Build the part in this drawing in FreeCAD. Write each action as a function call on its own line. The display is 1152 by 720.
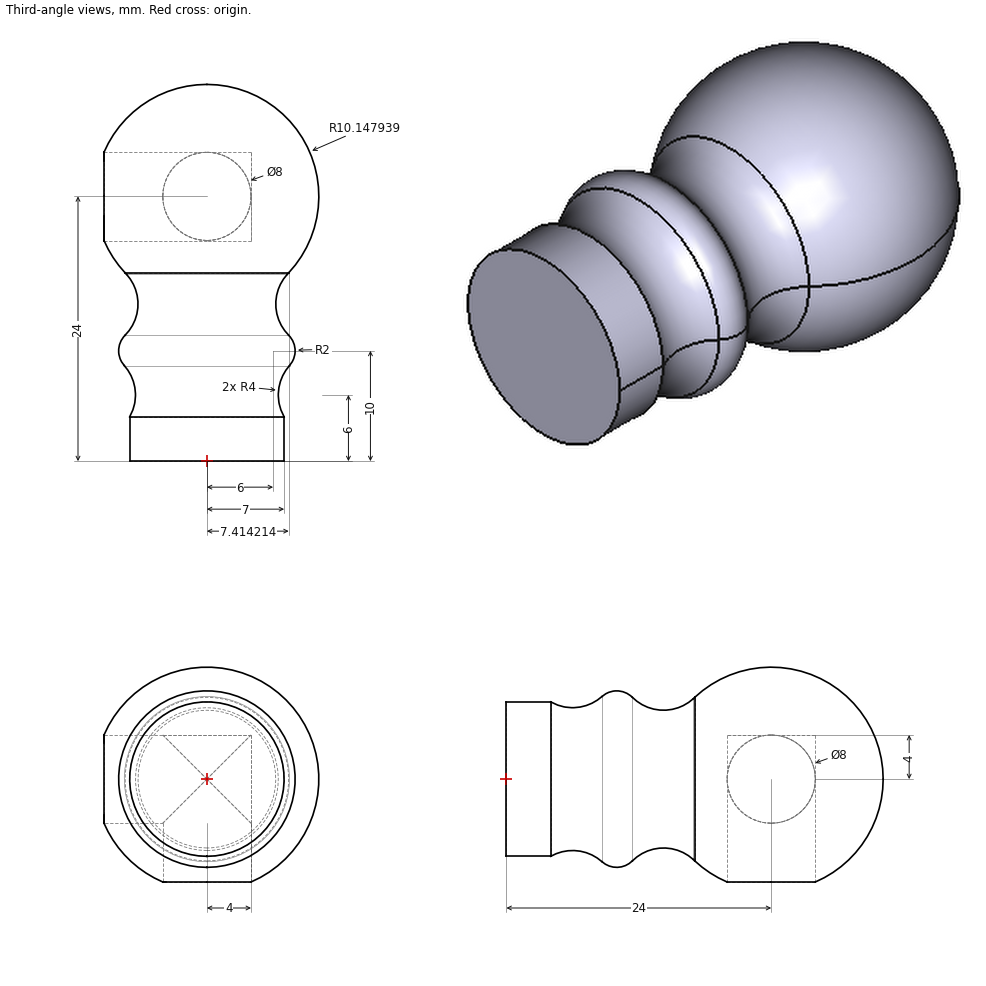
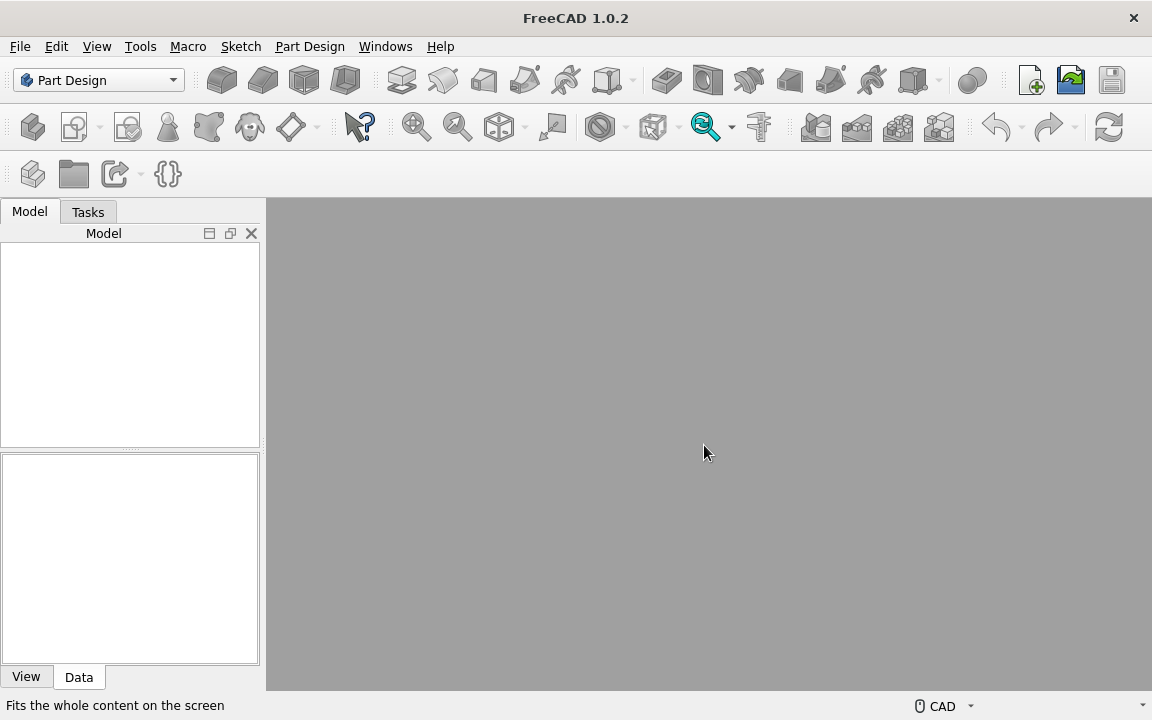
click(1030, 80)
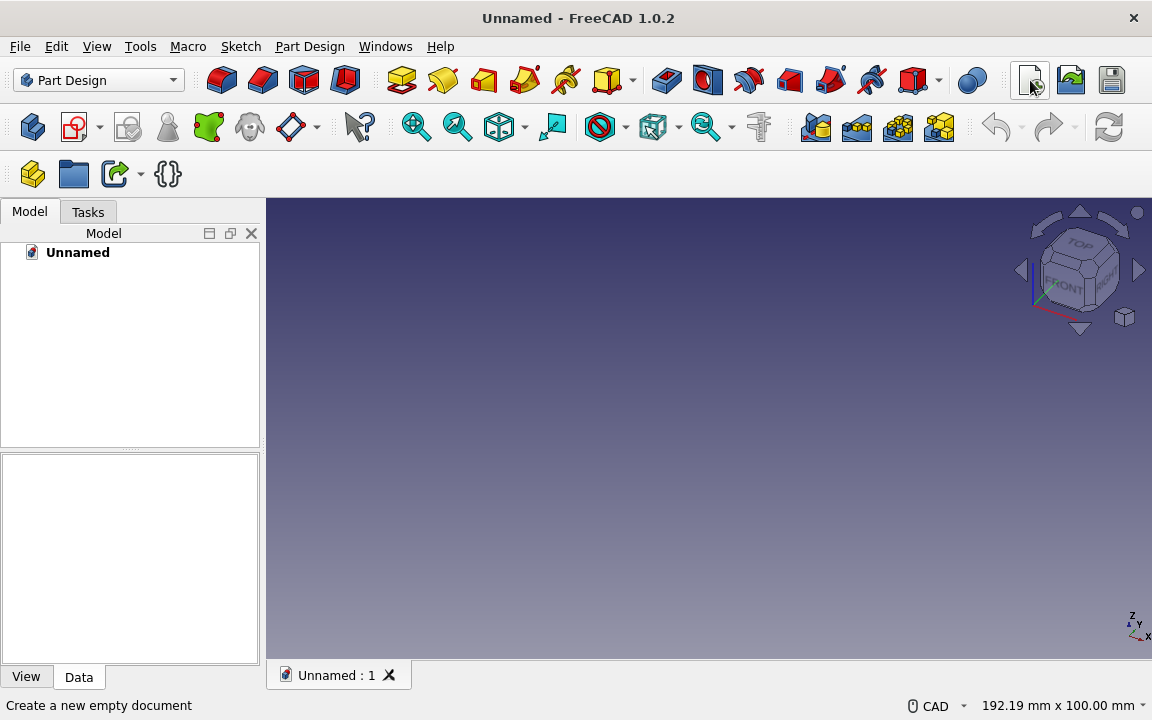
click(74, 128)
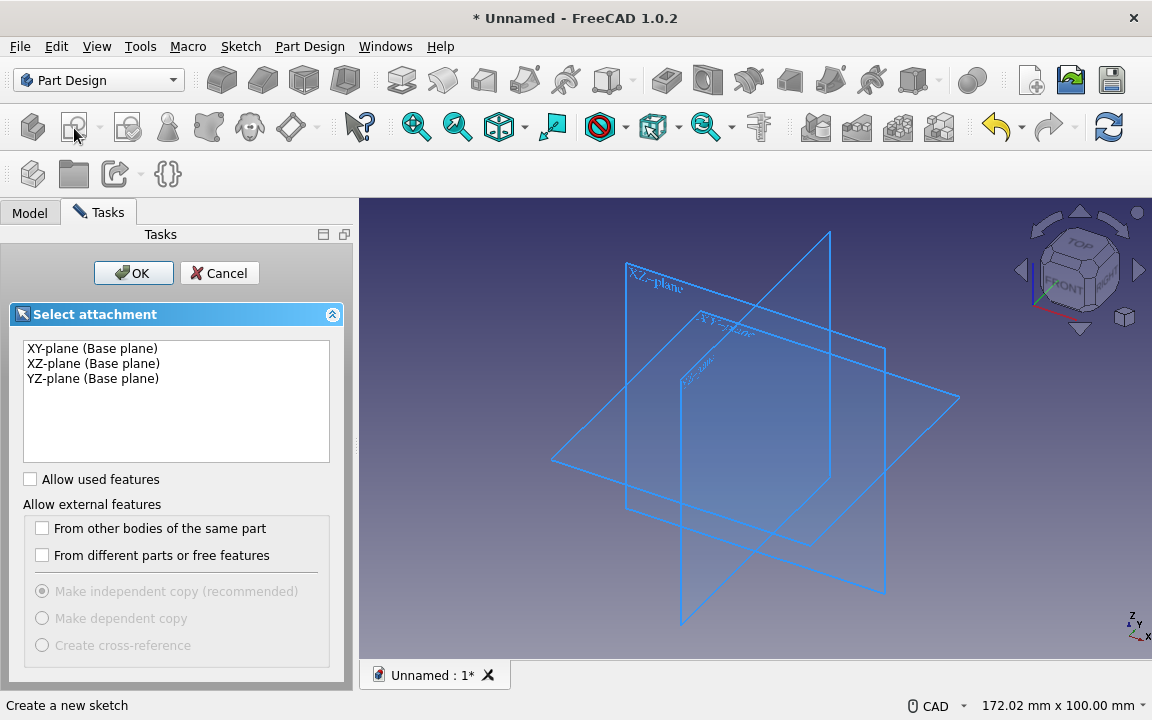
click(84, 348)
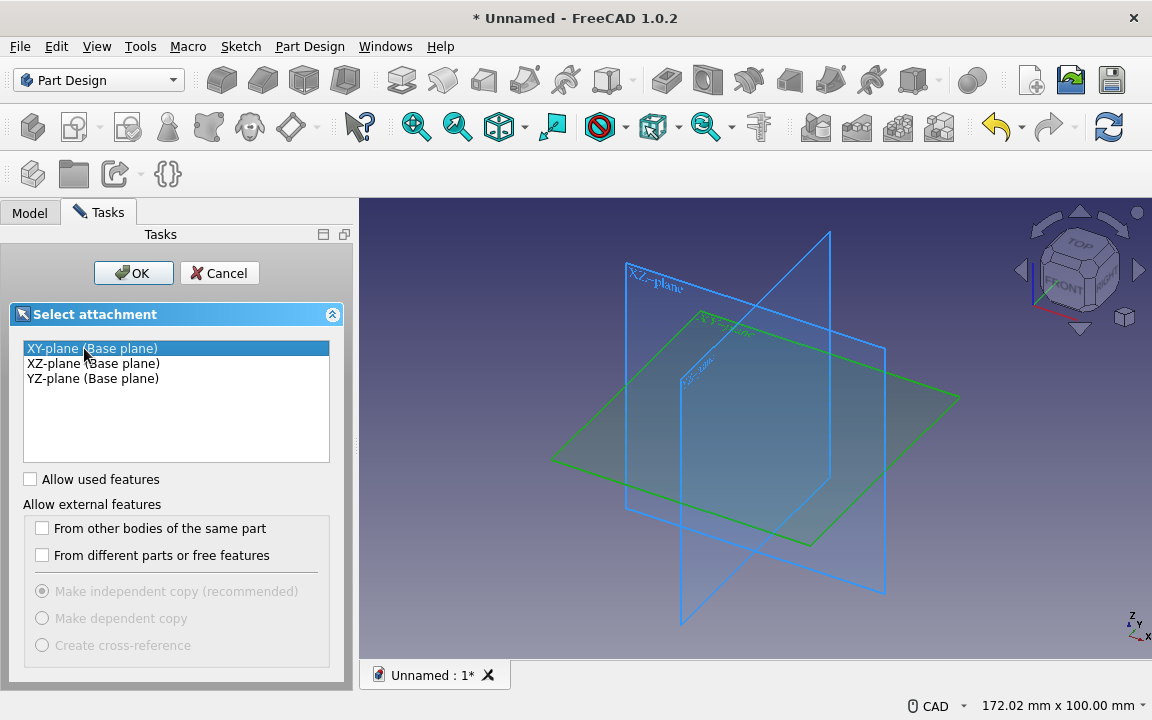
click(134, 273)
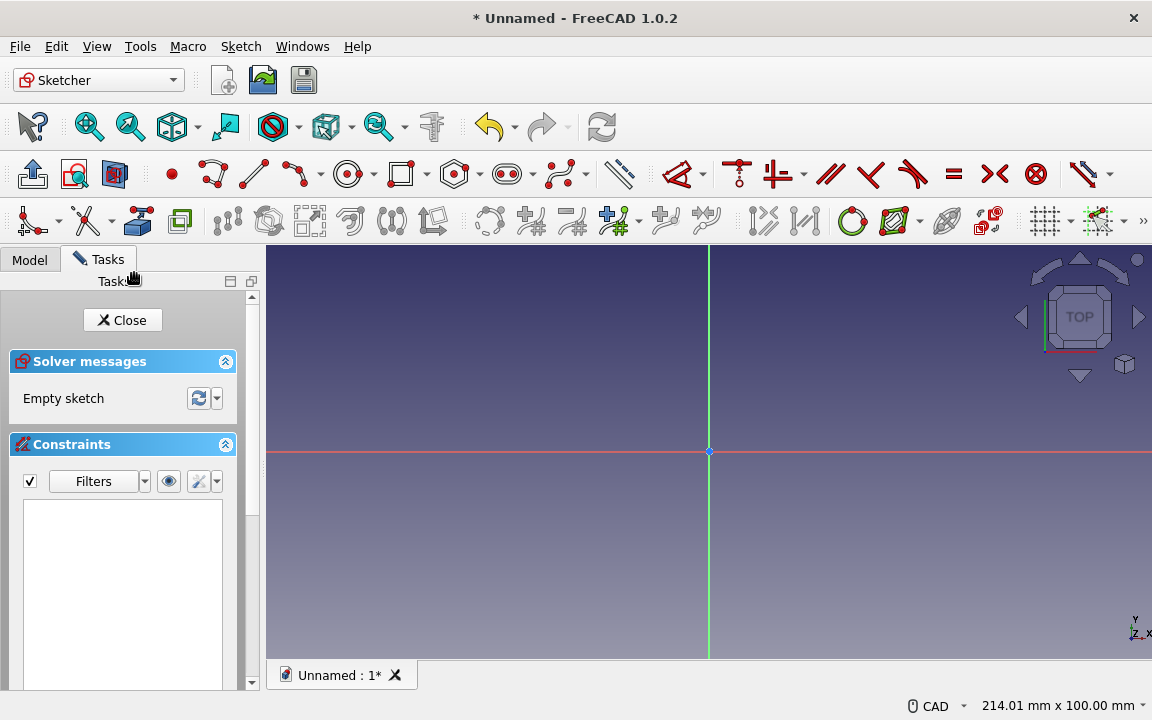
scroll(835, 295, up, 3)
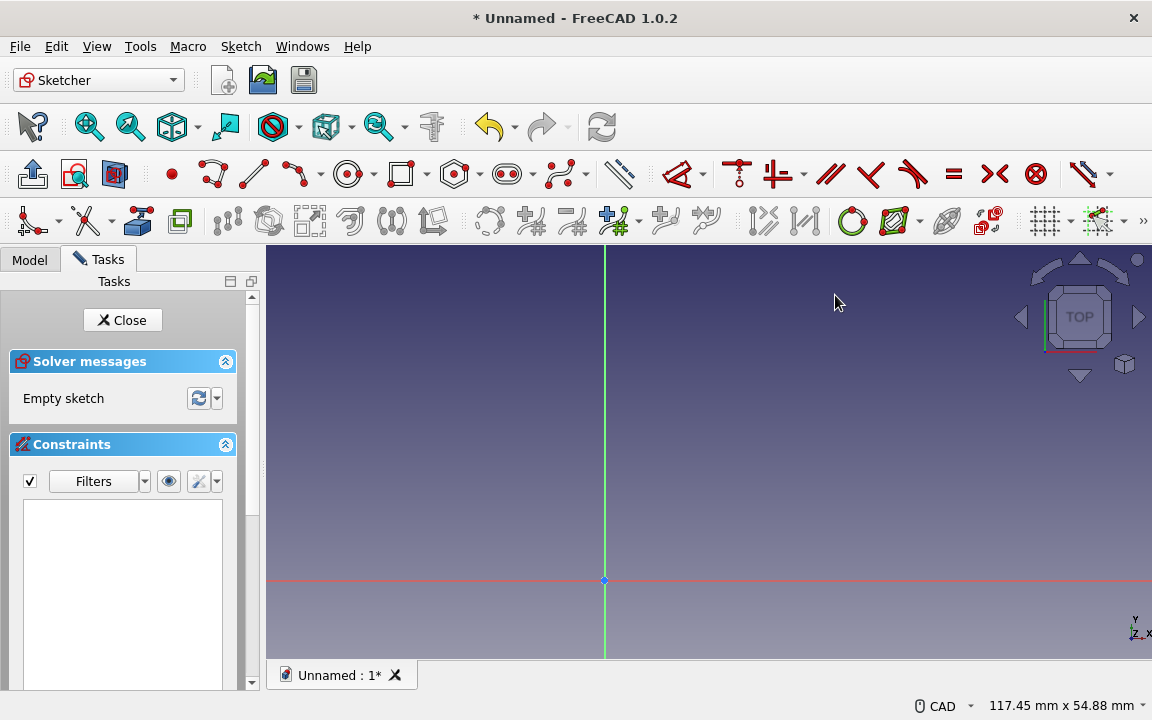
key(g)
key(m)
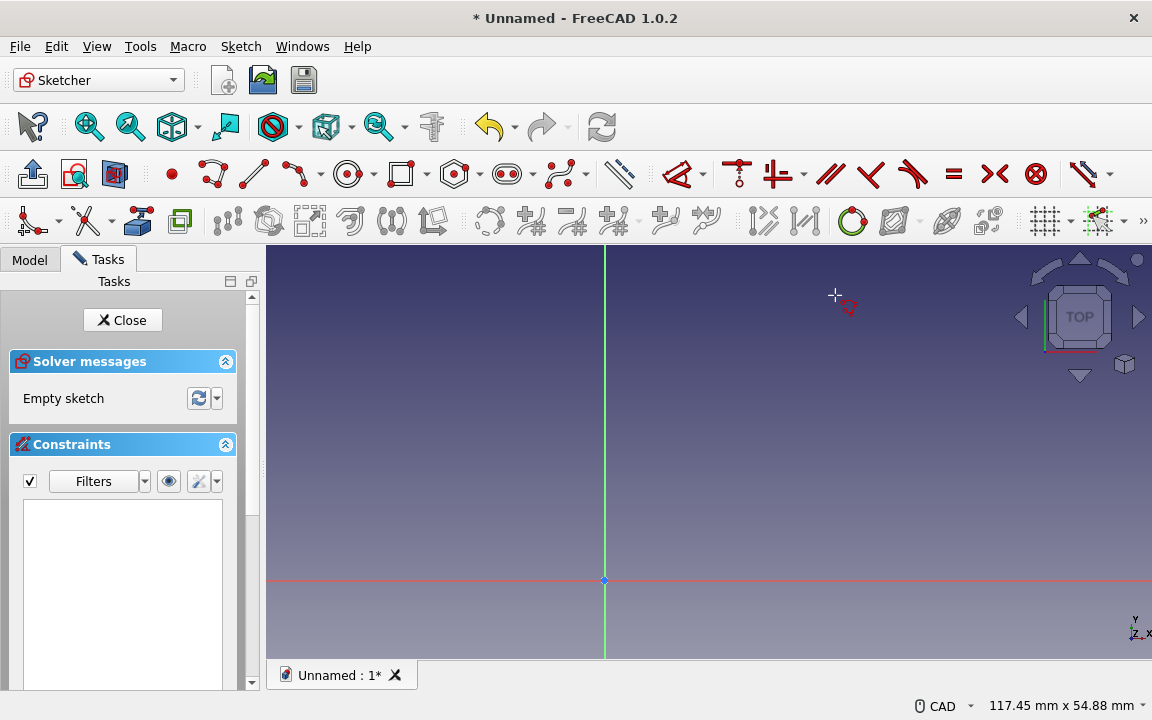
click(605, 323)
click(605, 581)
click(658, 572)
click(658, 551)
right_click(658, 551)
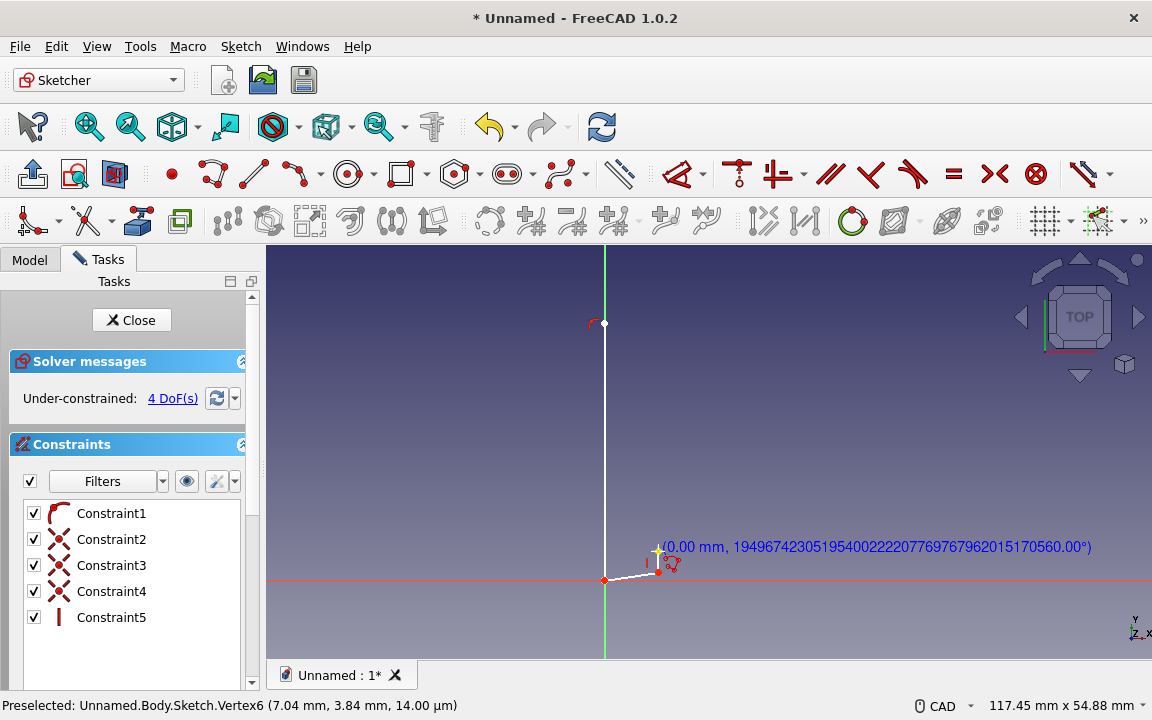
click(294, 174)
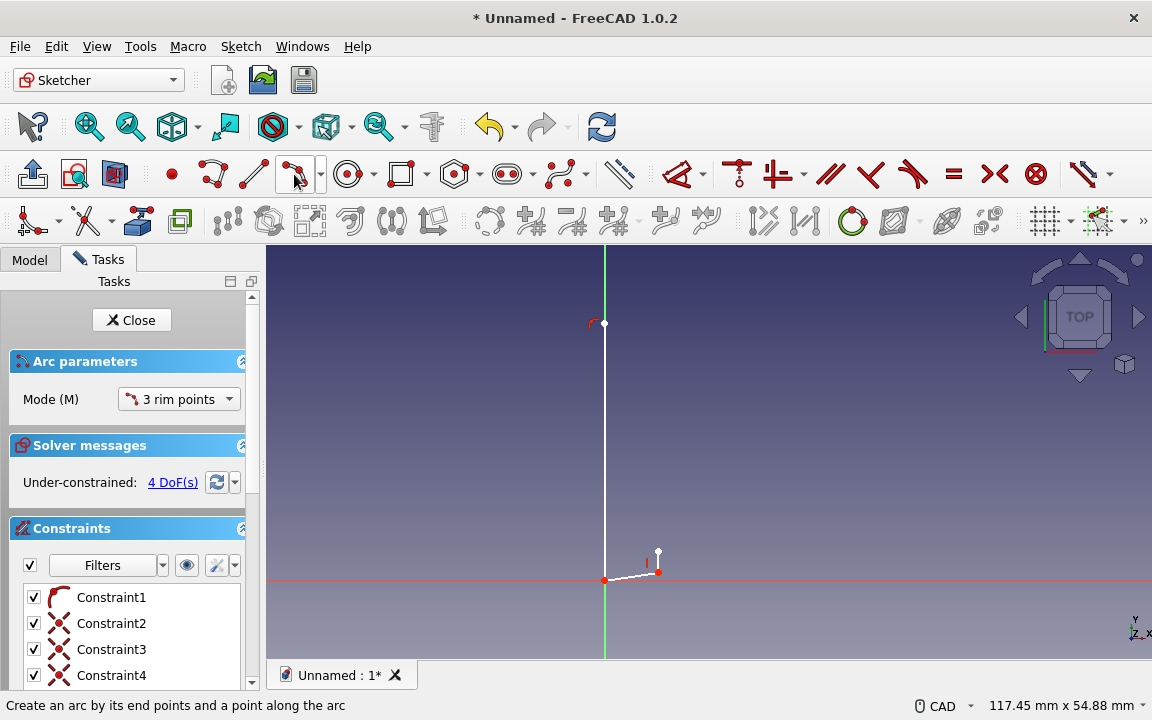
click(658, 552)
click(661, 516)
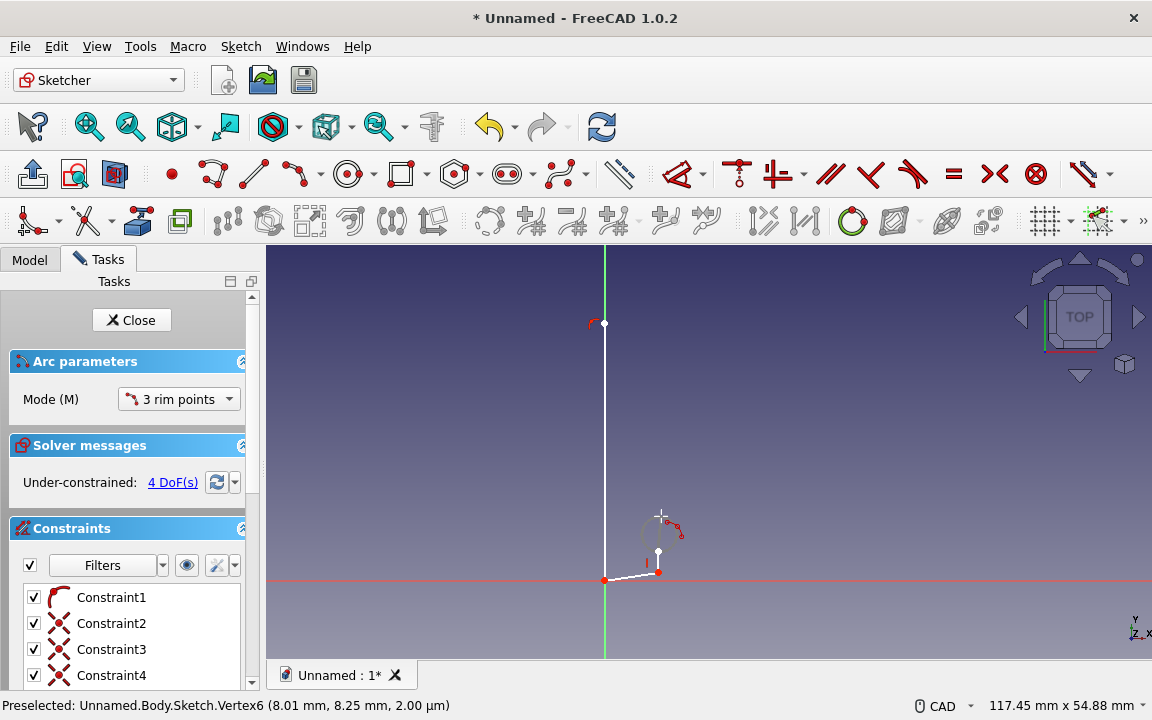
scroll(654, 533, up, 6)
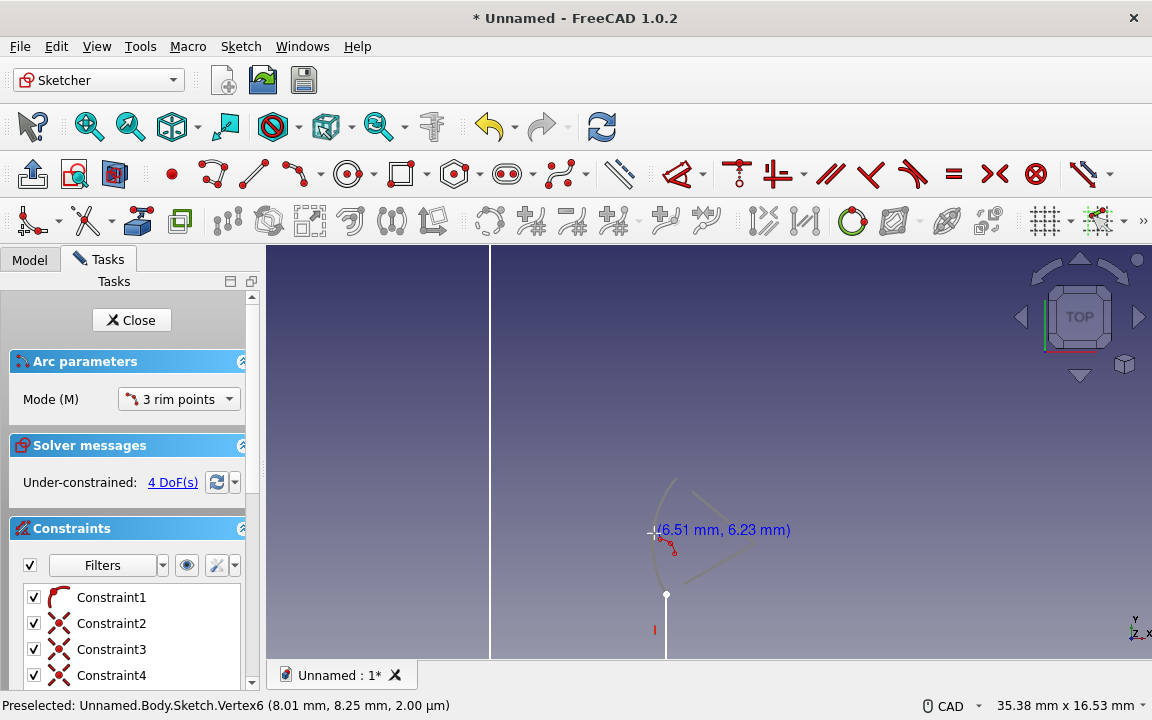
click(653, 530)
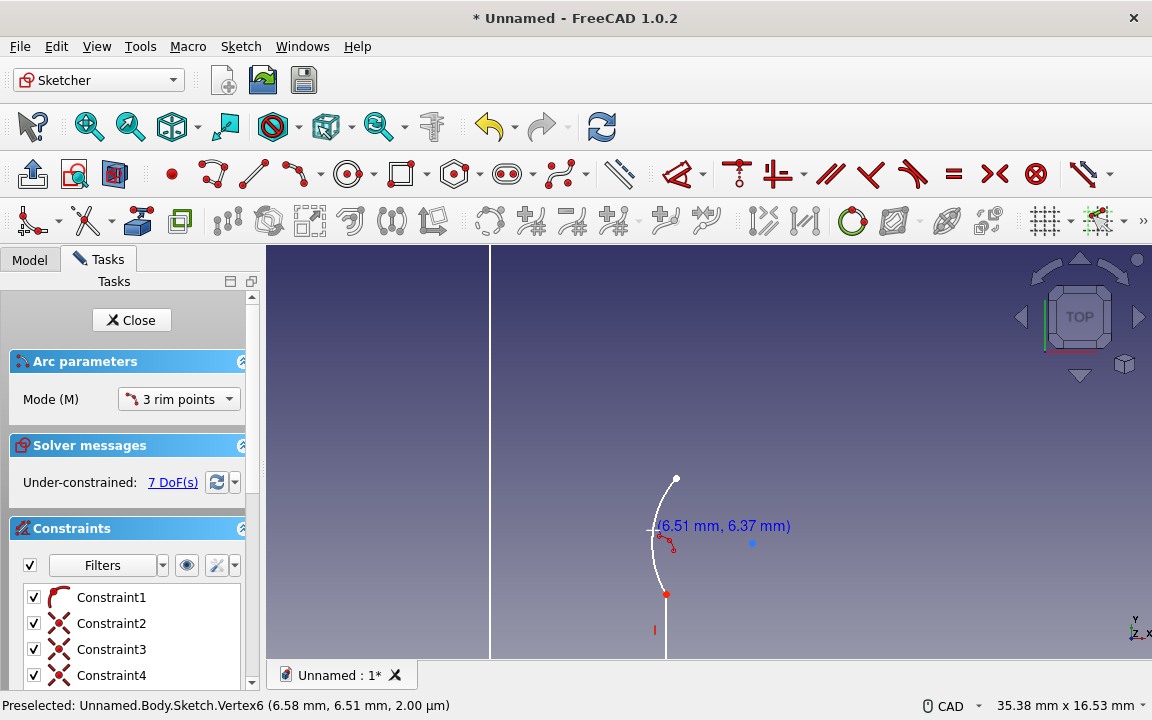
click(676, 478)
click(676, 405)
click(690, 439)